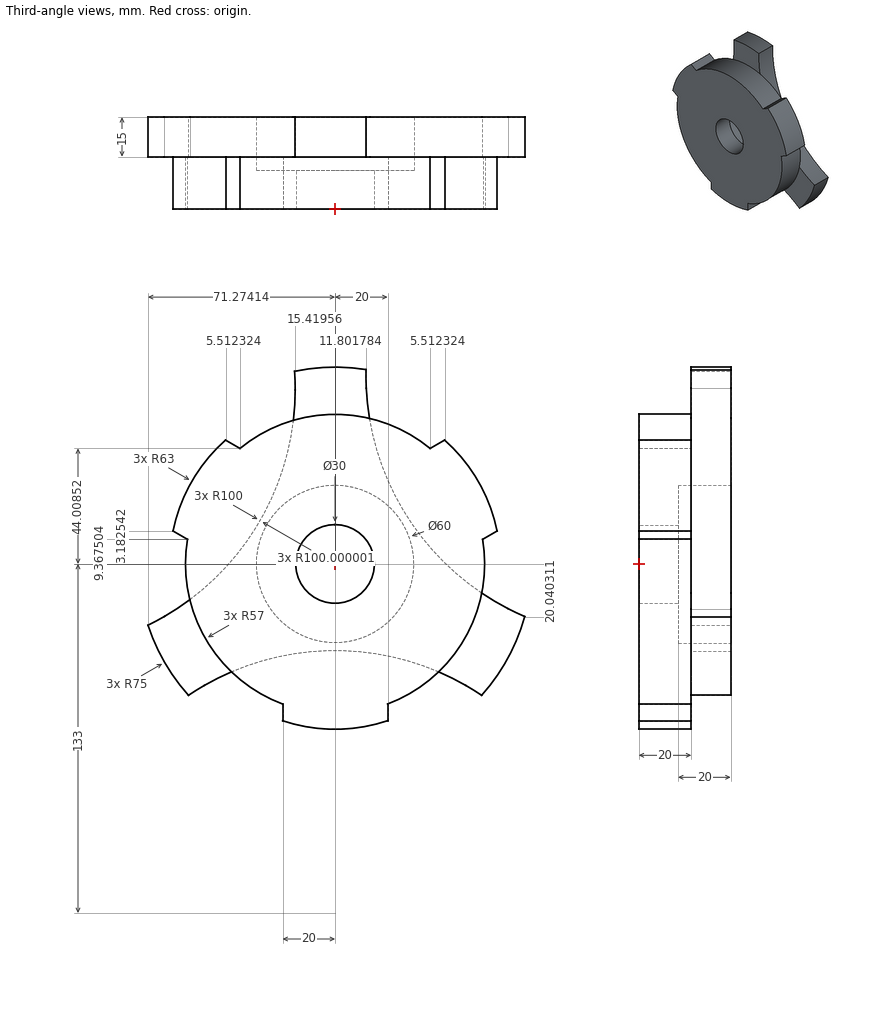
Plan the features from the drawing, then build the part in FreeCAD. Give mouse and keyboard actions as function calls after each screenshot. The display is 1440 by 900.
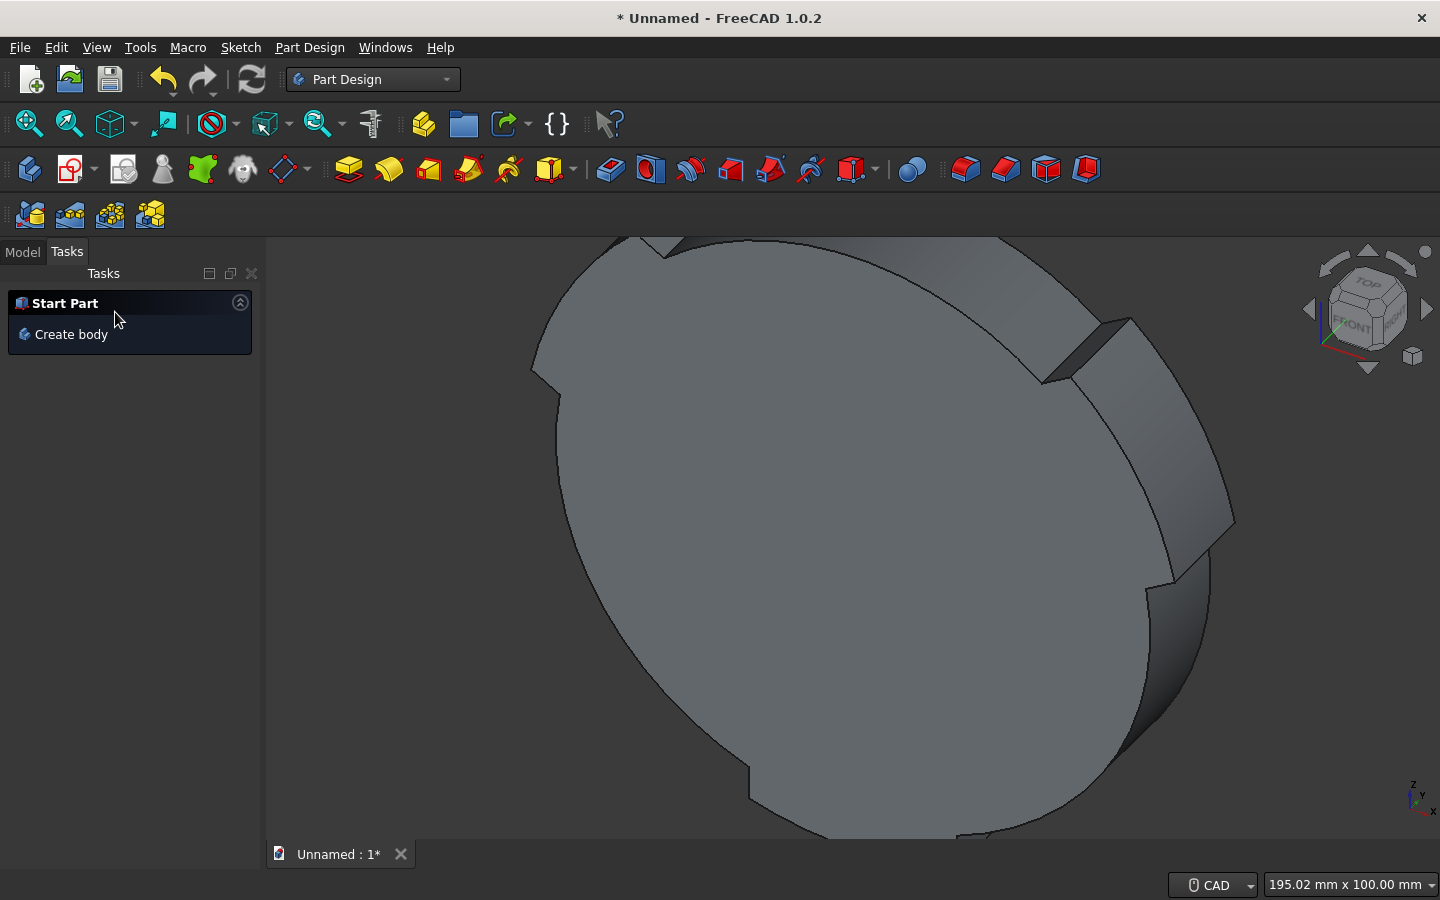
click(30, 124)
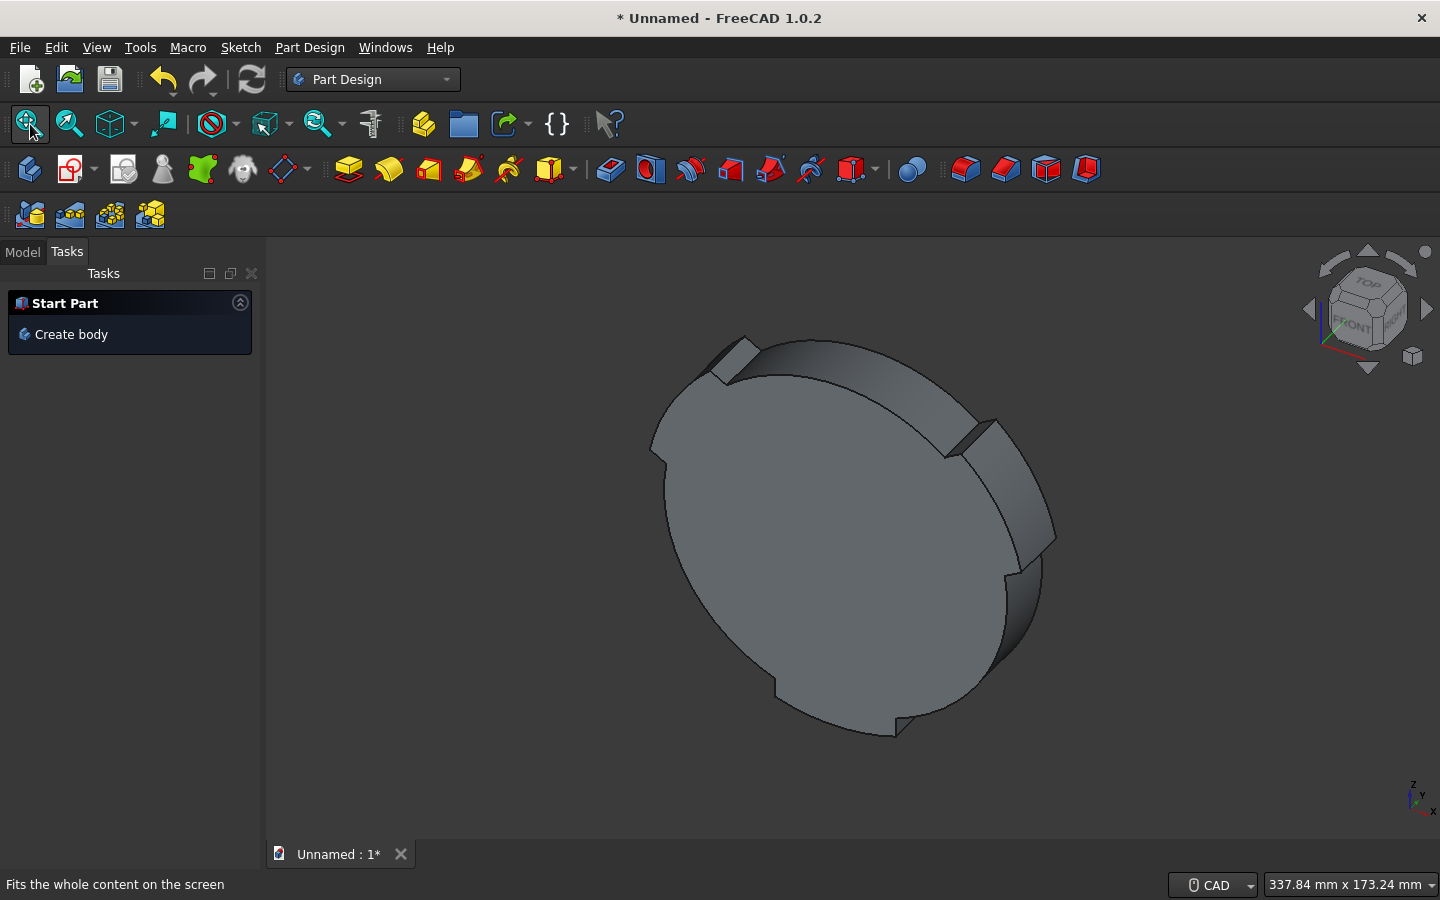
key(4)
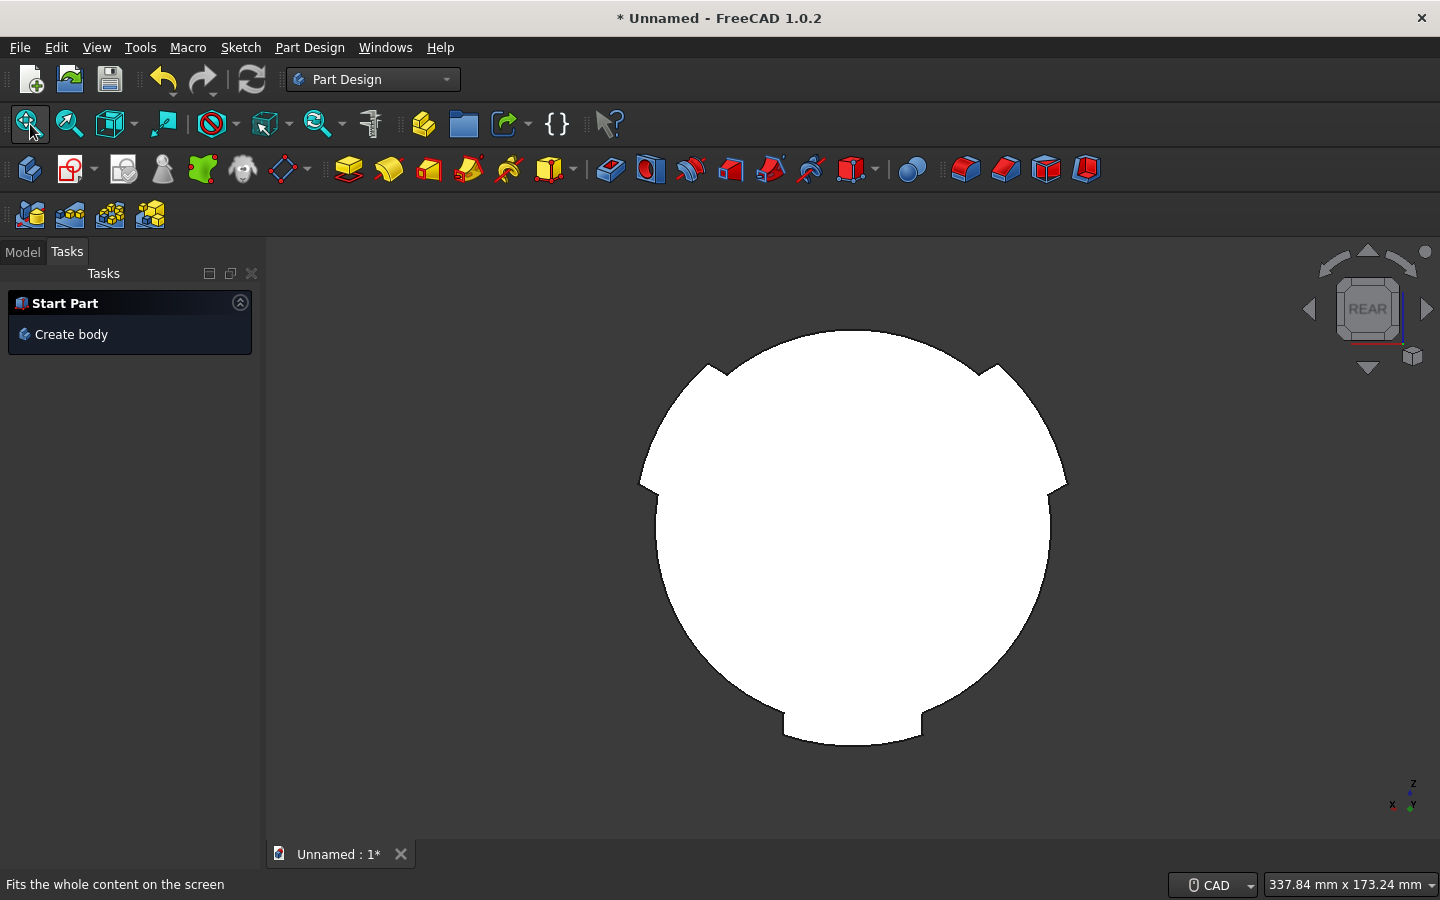
click(853, 537)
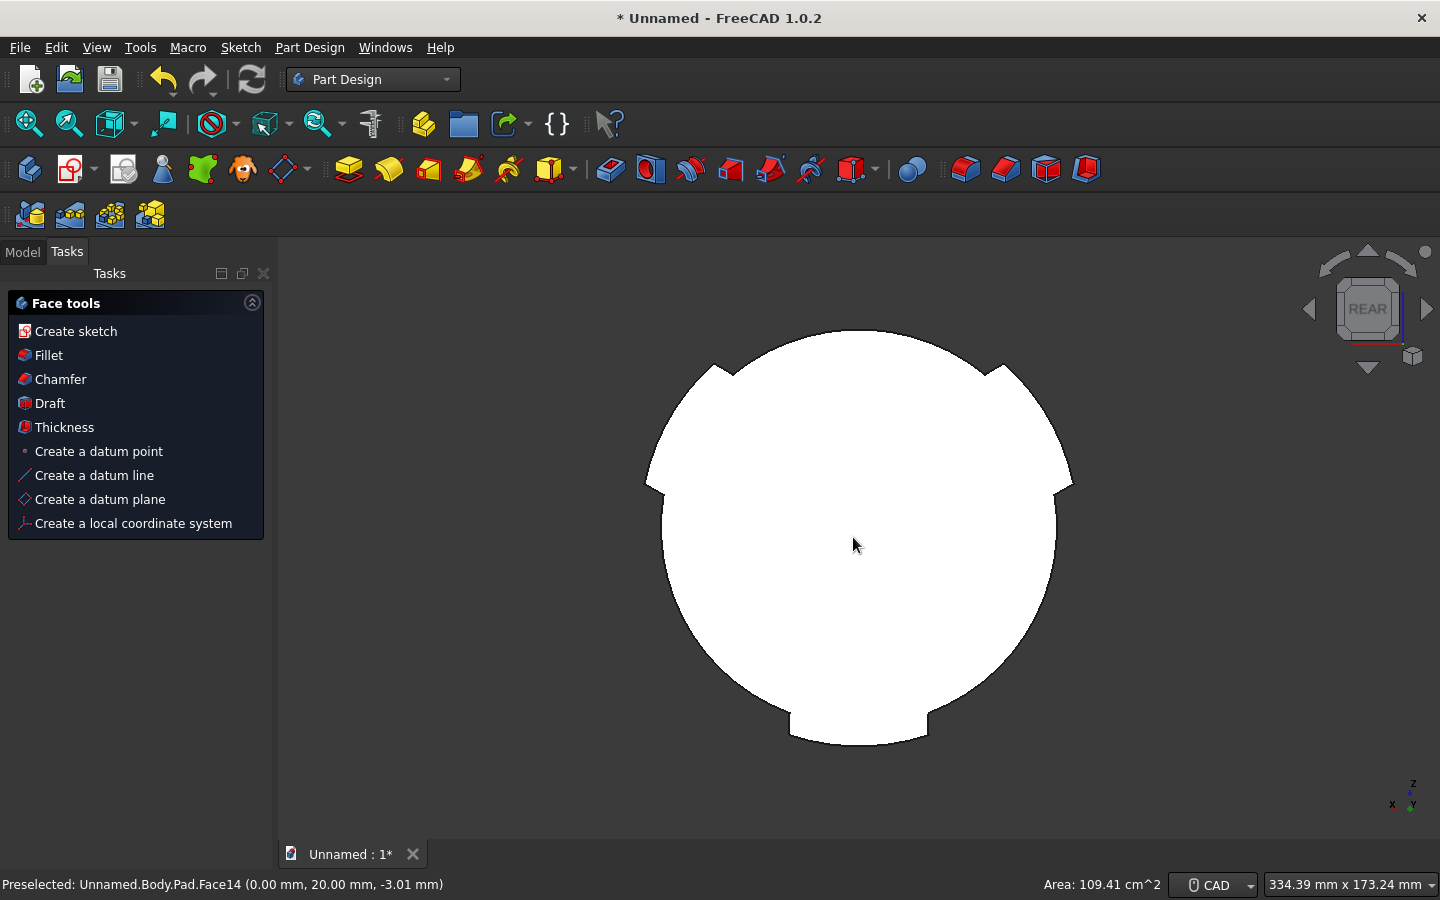
click(70, 170)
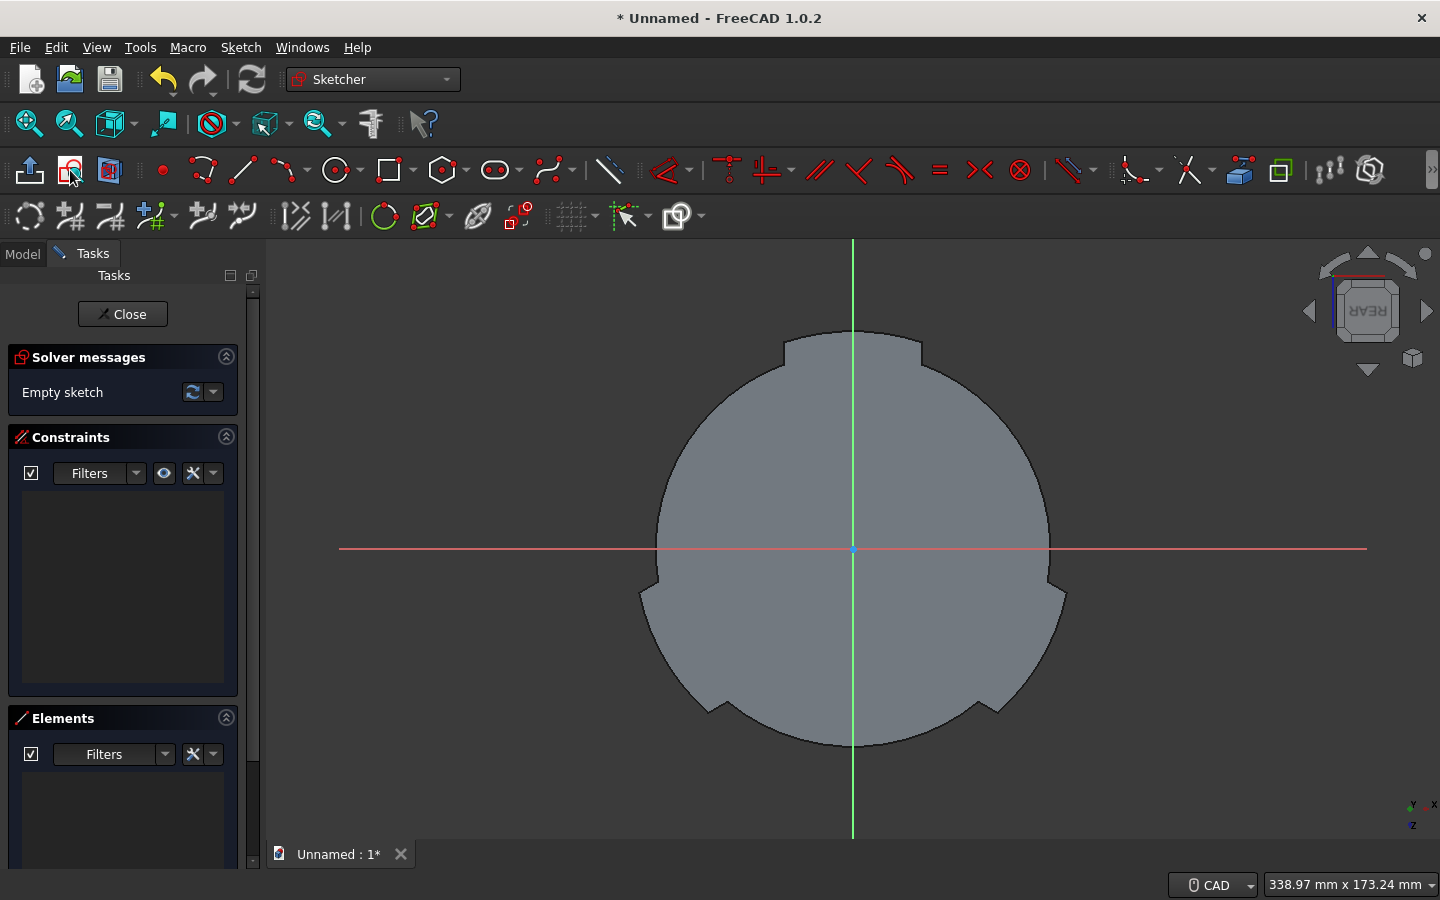
scroll(467, 297, down, 1)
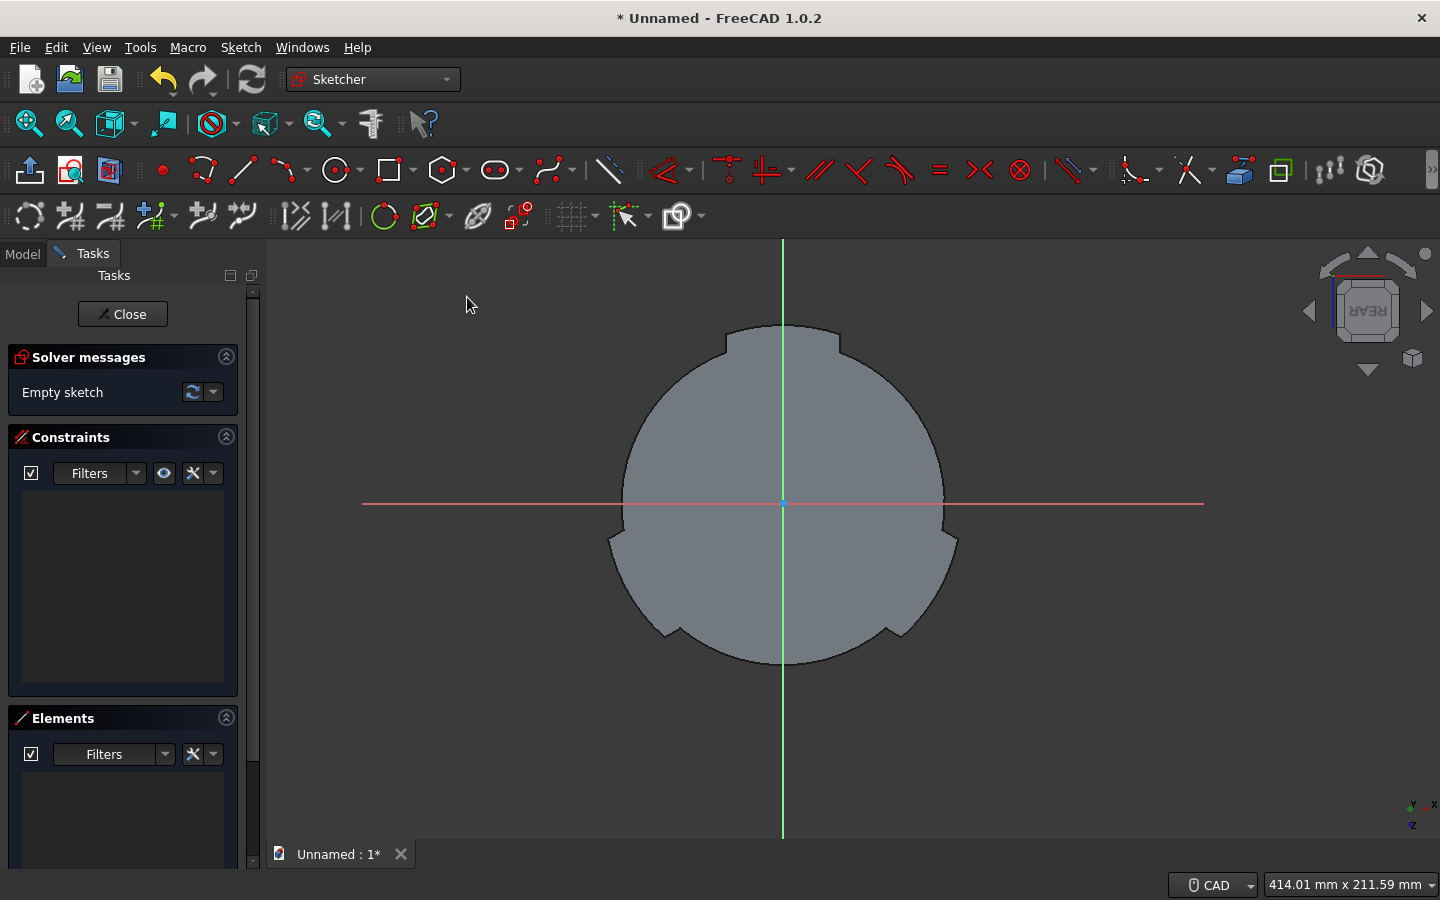
click(284, 170)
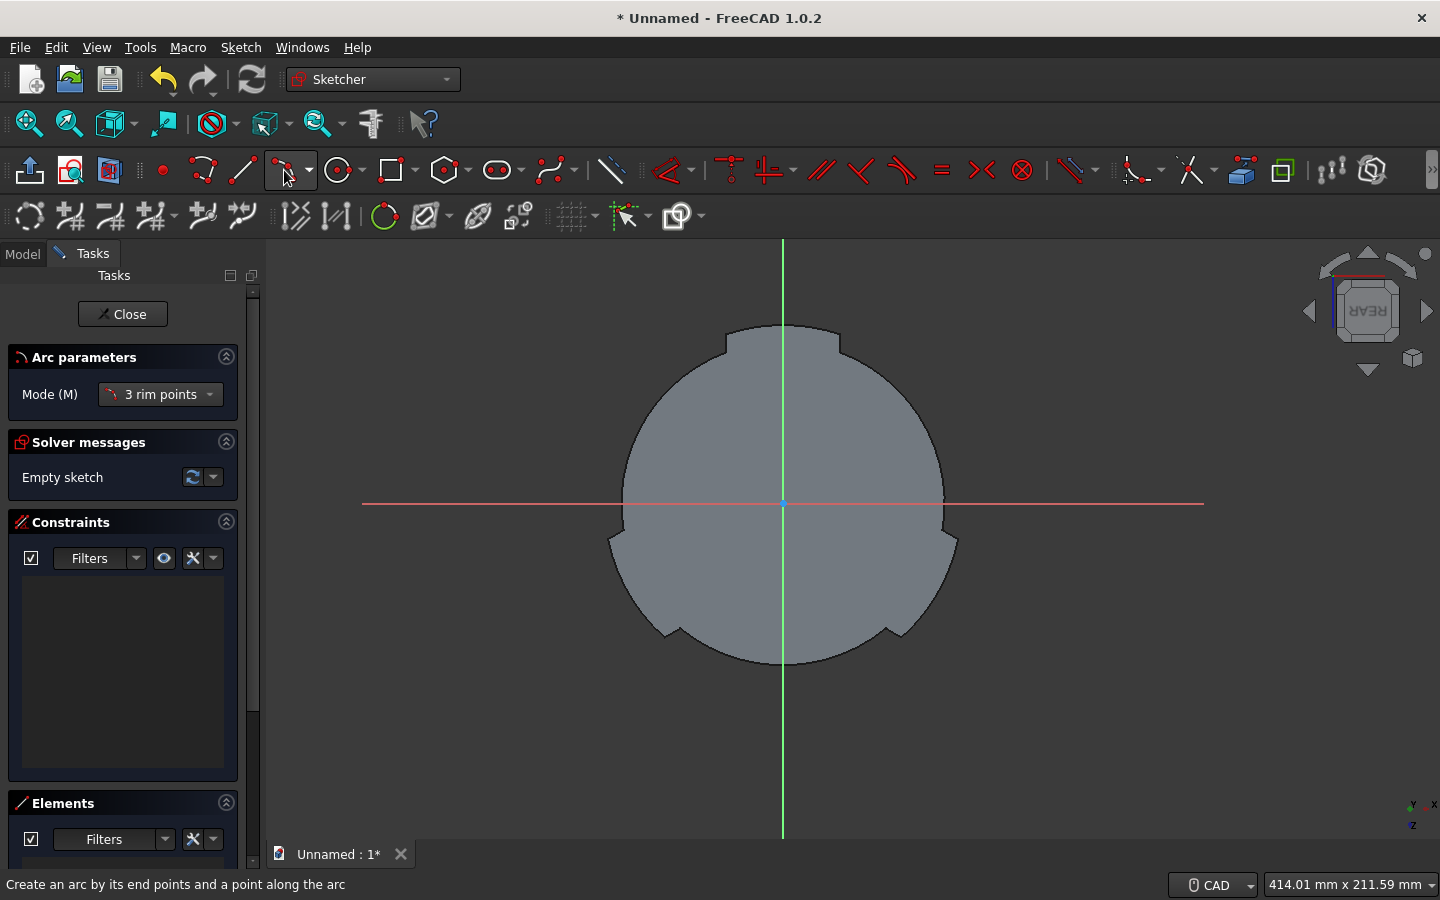
click(581, 437)
click(739, 712)
click(702, 550)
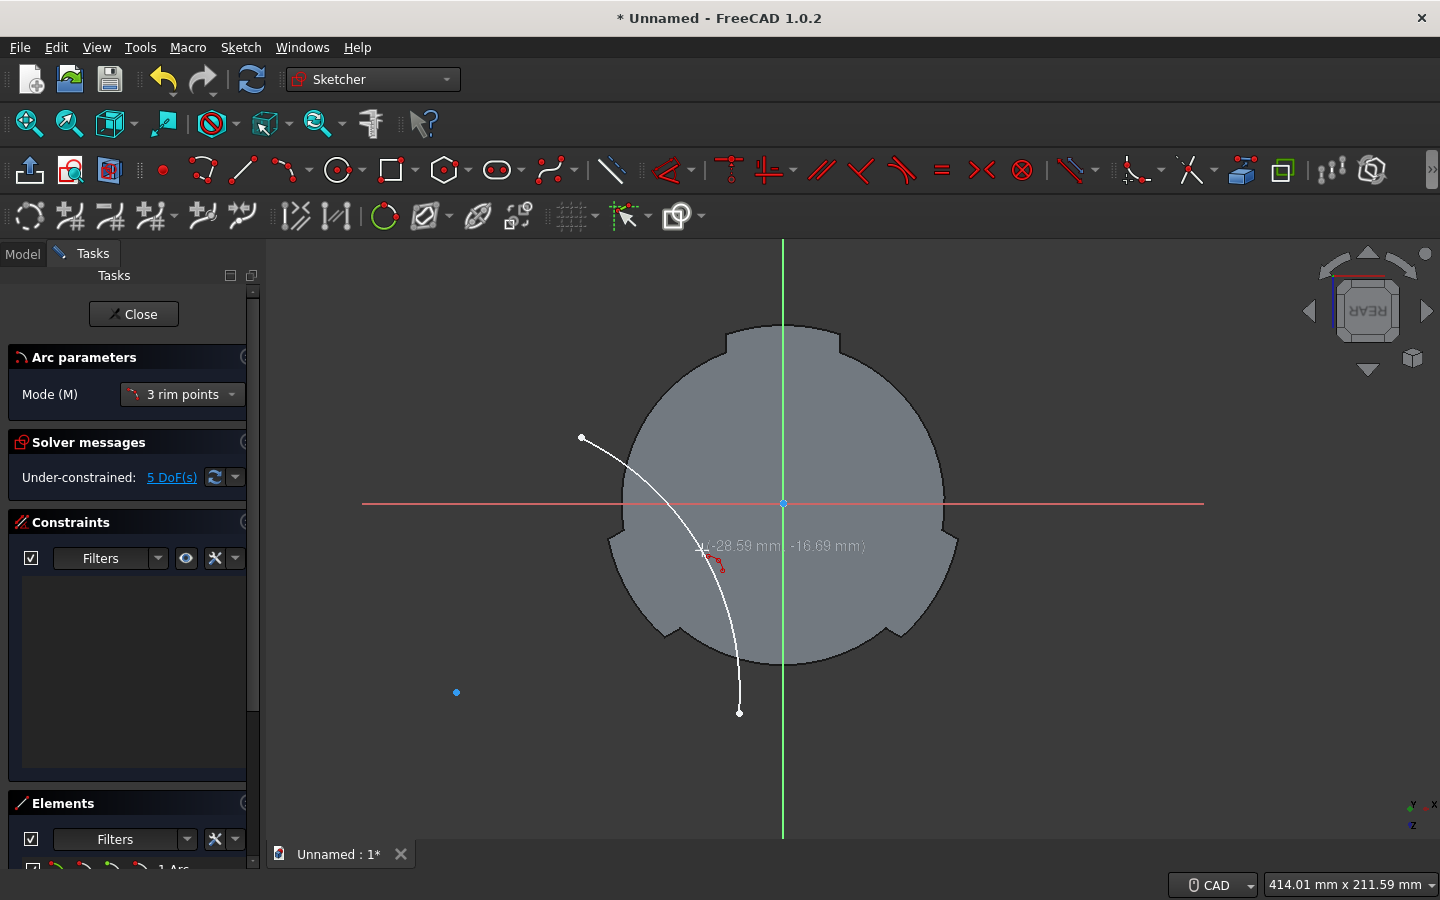
click(739, 713)
click(817, 714)